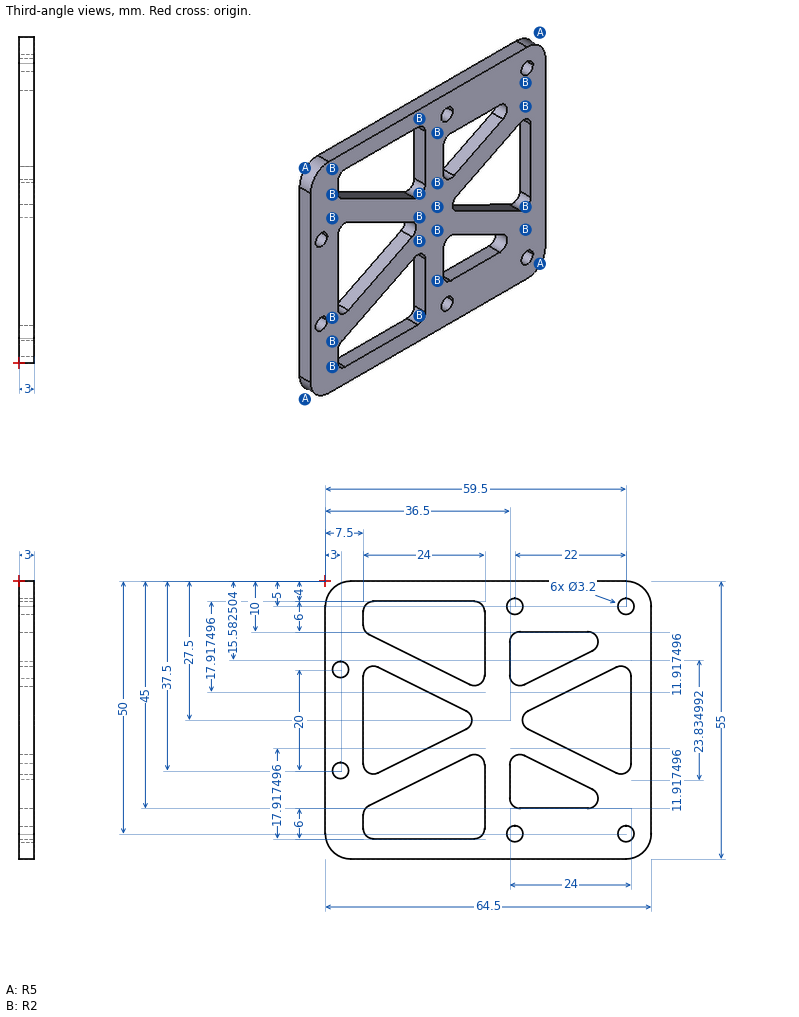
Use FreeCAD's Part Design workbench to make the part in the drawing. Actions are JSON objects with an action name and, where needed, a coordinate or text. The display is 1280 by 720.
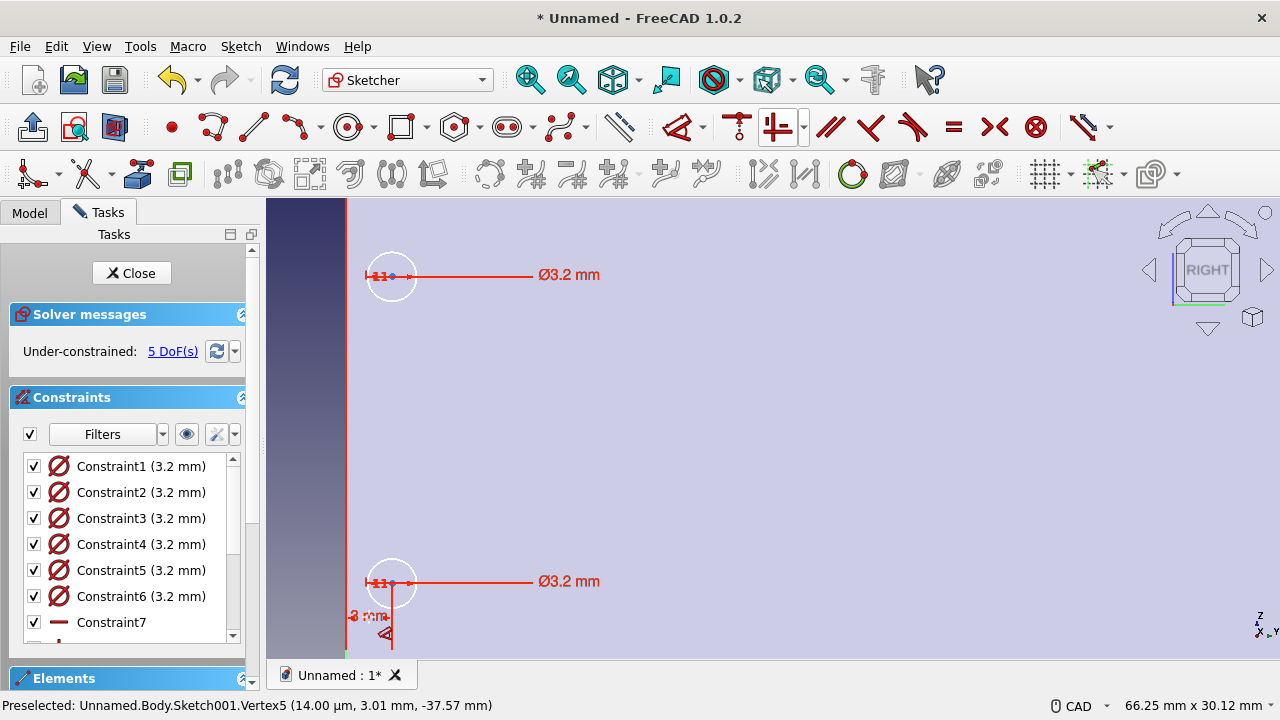
{"action": "scroll", "coordinate": [641, 443], "scroll_direction": "down", "scroll_amount": 5}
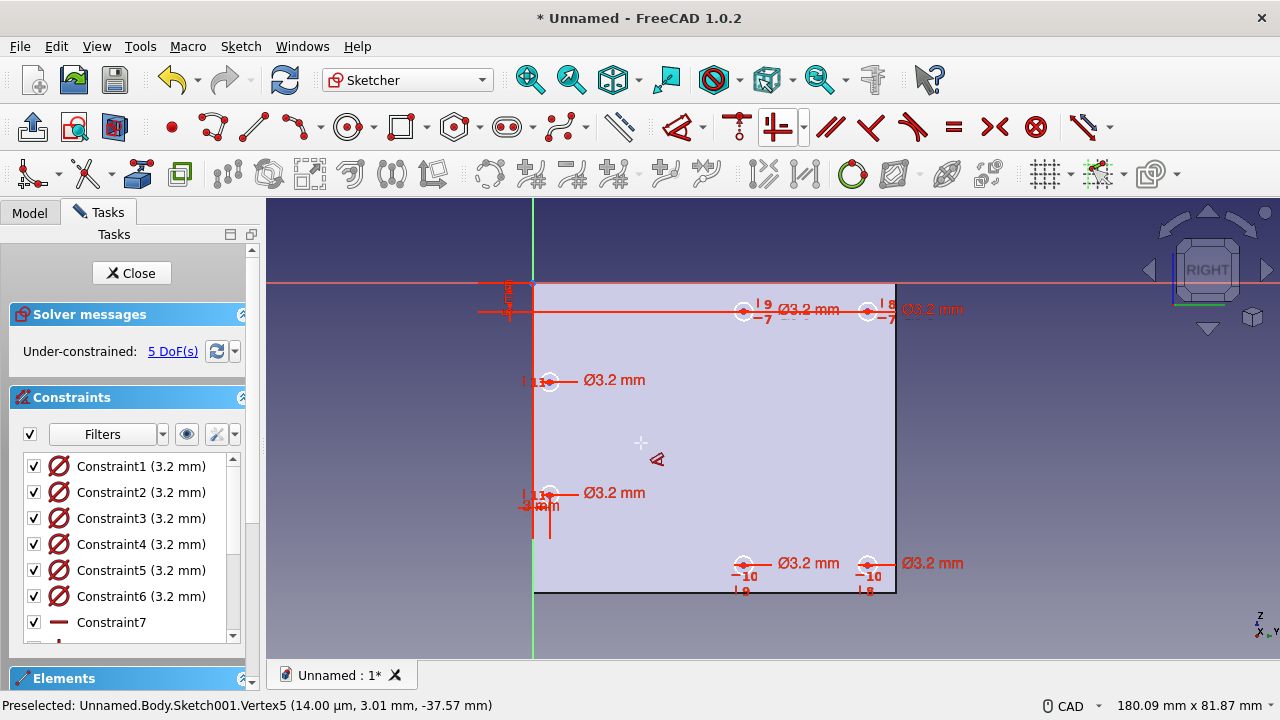
{"action": "left_click", "coordinate": [868, 565]}
{"action": "left_click", "coordinate": [499, 424]}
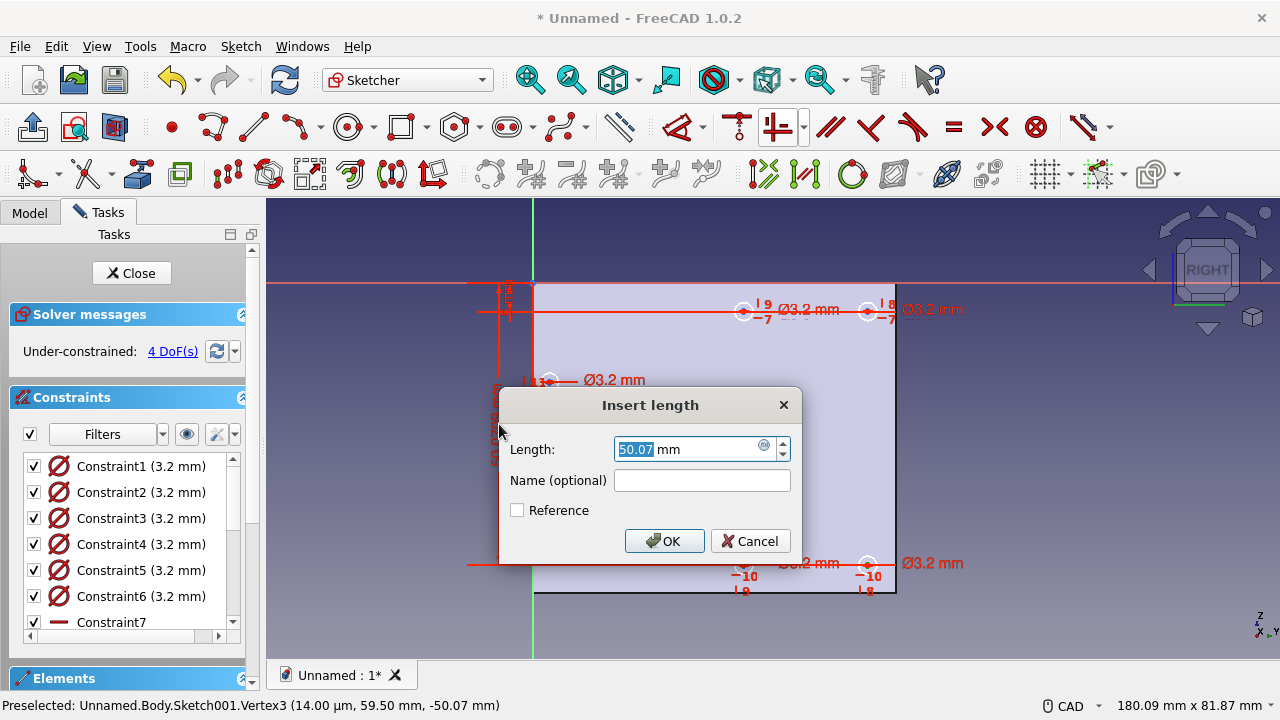
{"action": "type", "text": "50"}
{"action": "key", "text": "Return"}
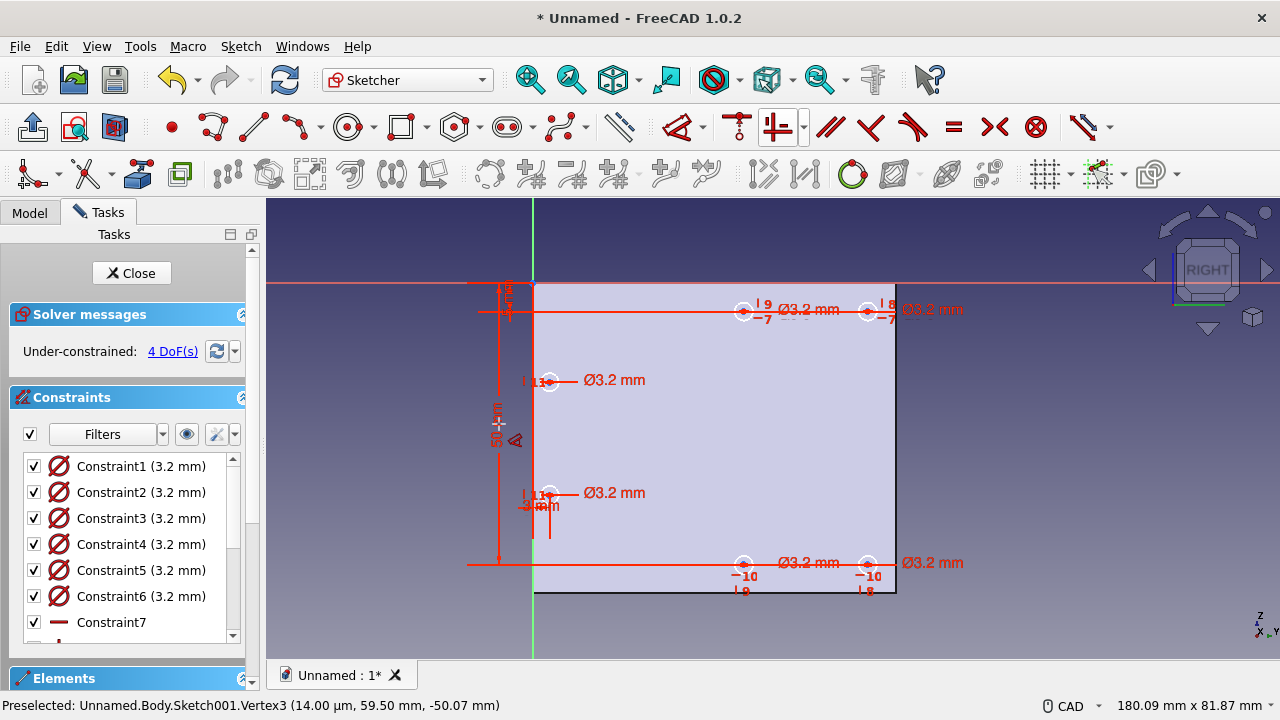
{"action": "left_click", "coordinate": [868, 312]}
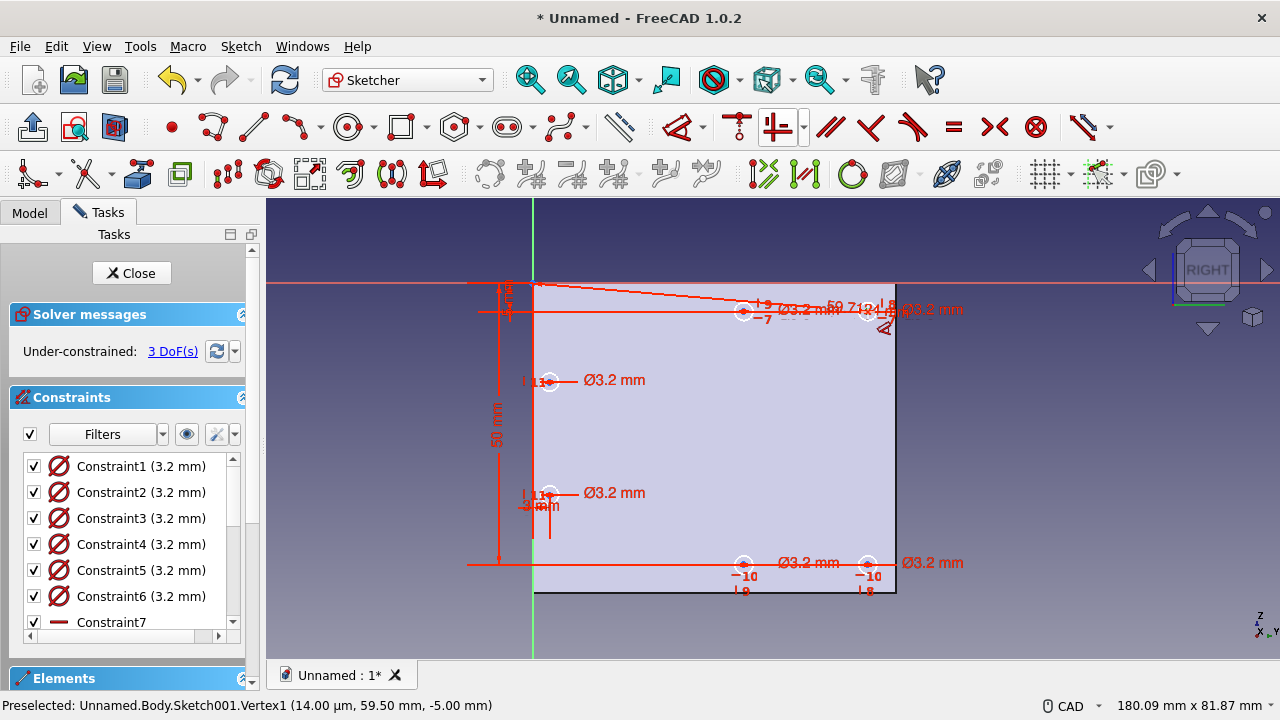
{"action": "left_click", "coordinate": [744, 312]}
{"action": "left_click", "coordinate": [806, 346]}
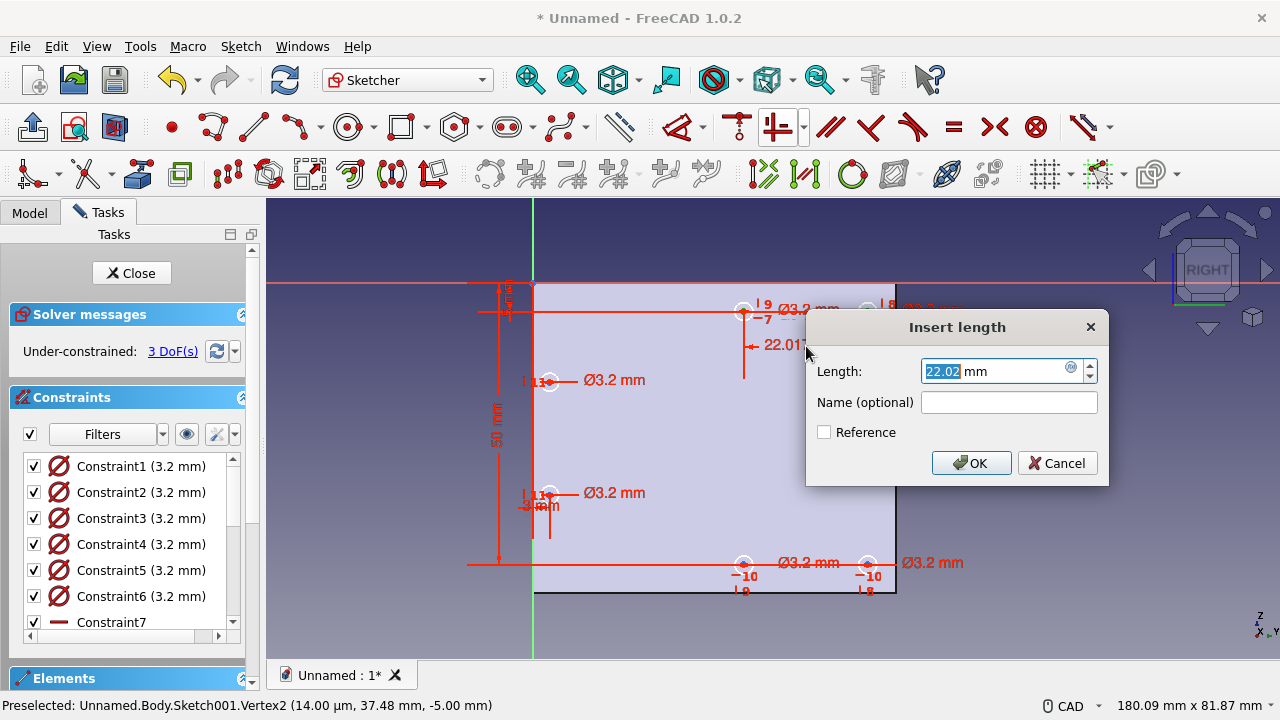
{"action": "type", "text": "22"}
{"action": "key", "text": "Return"}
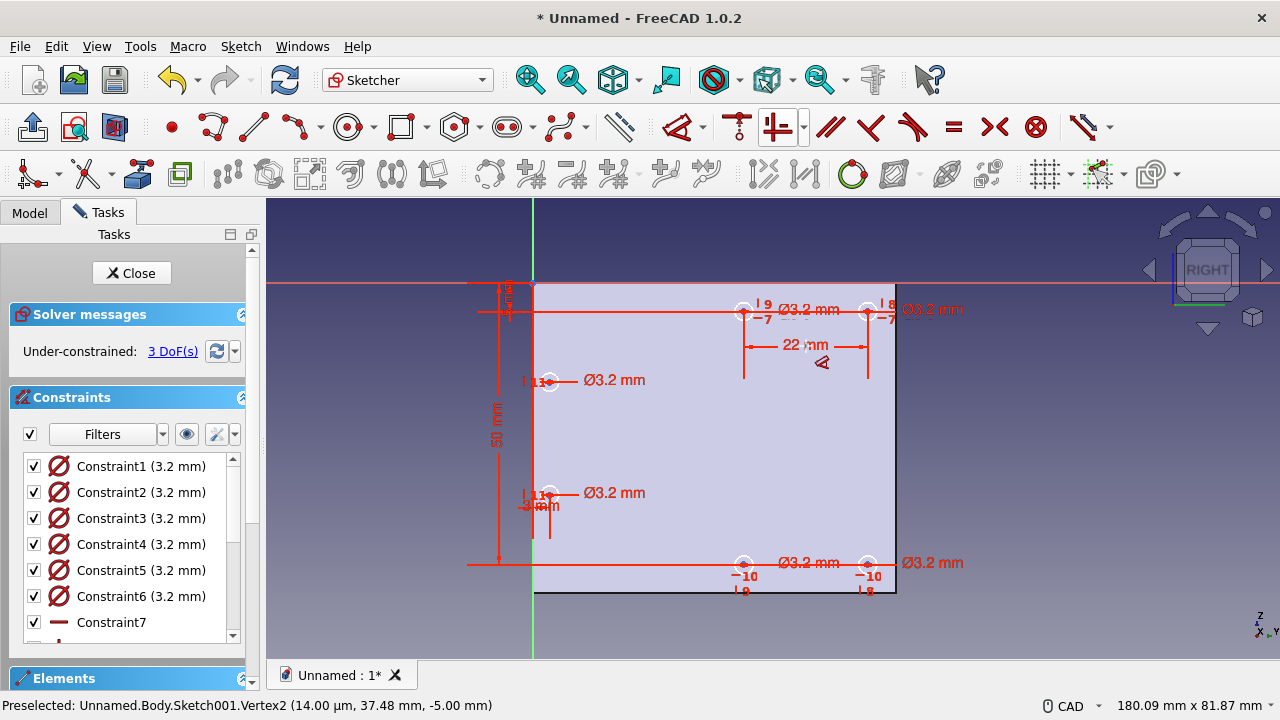
{"action": "left_click", "coordinate": [550, 495]}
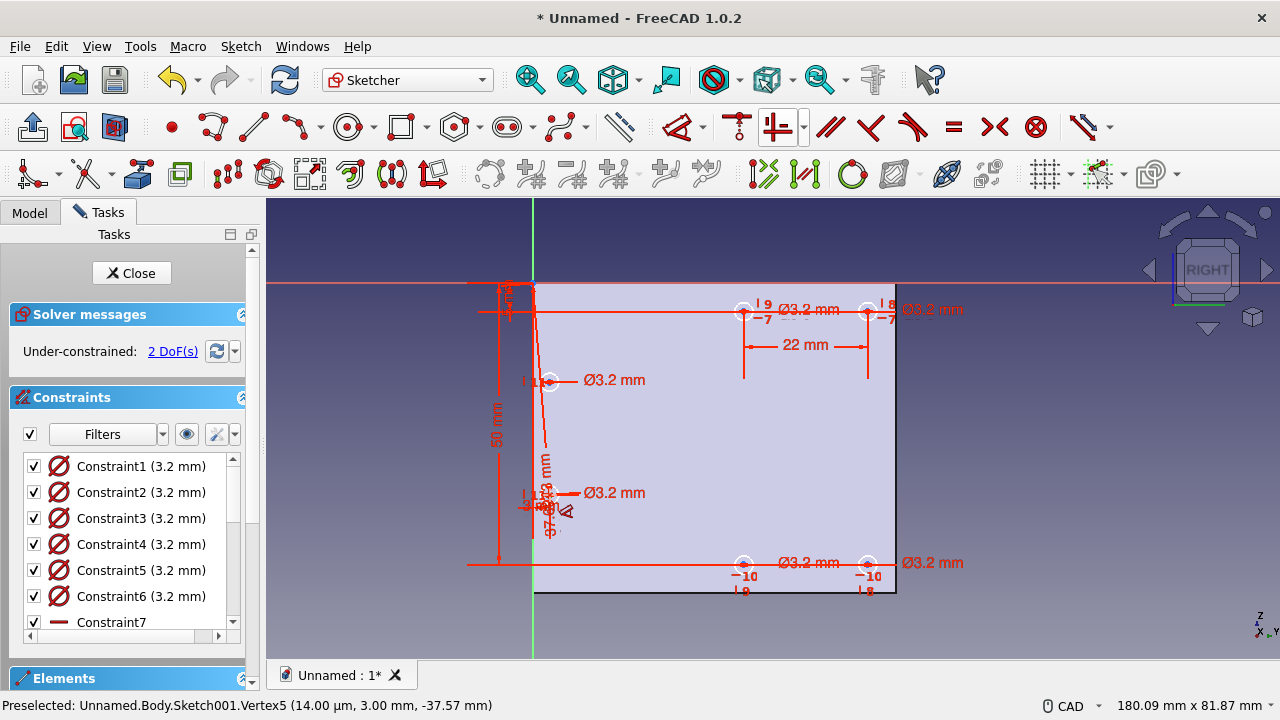
{"action": "left_click", "coordinate": [550, 382]}
{"action": "left_click", "coordinate": [516, 465]}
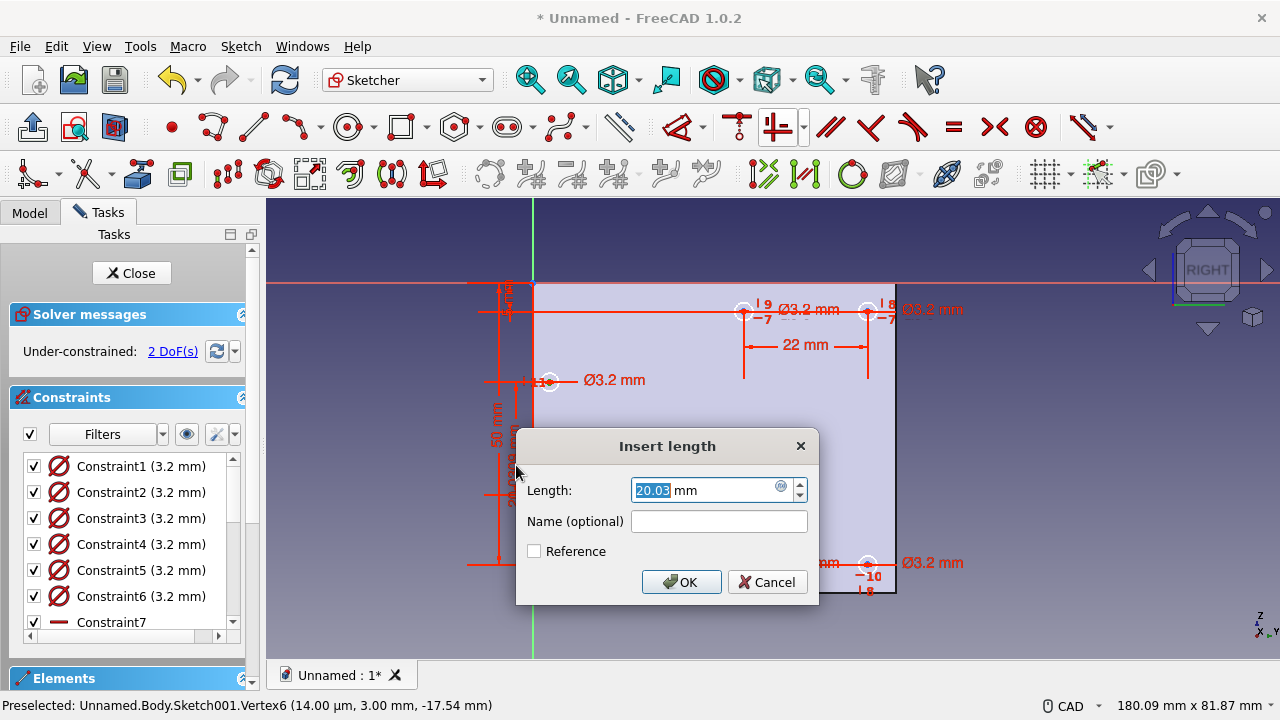
{"action": "type", "text": "20"}
{"action": "key", "text": "Return"}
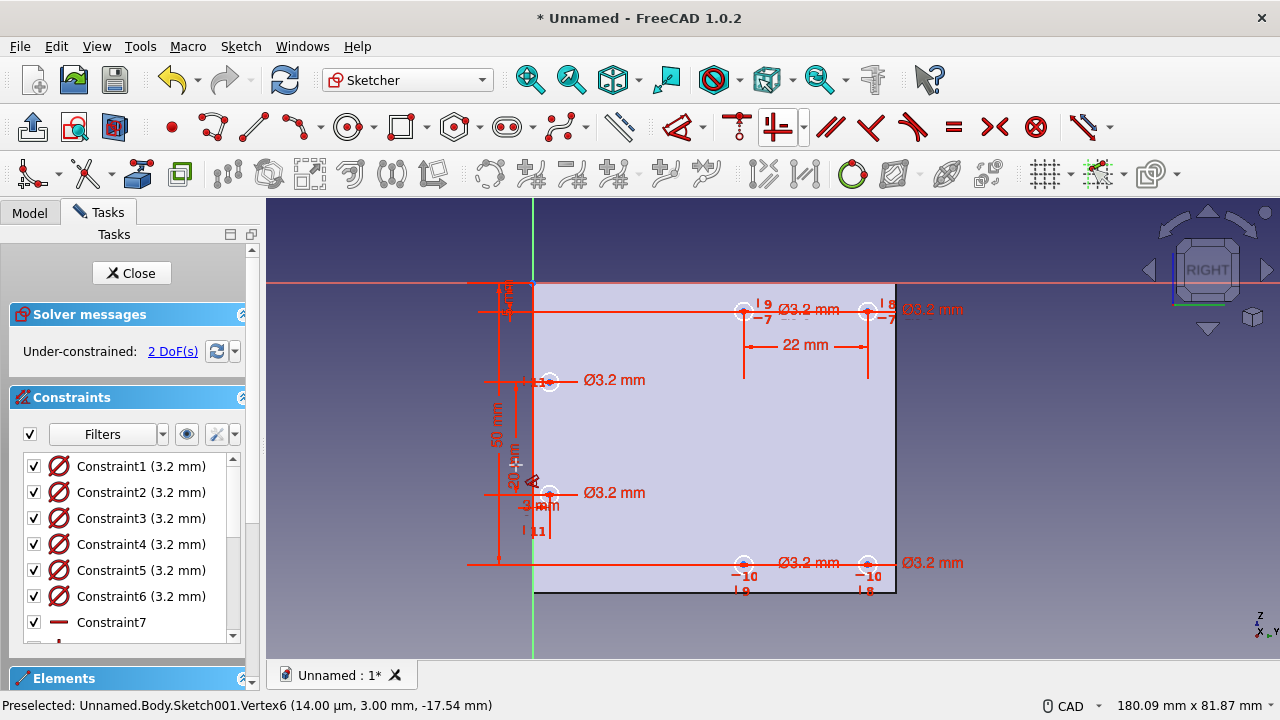
{"action": "left_click", "coordinate": [868, 312]}
{"action": "left_click", "coordinate": [700, 249]}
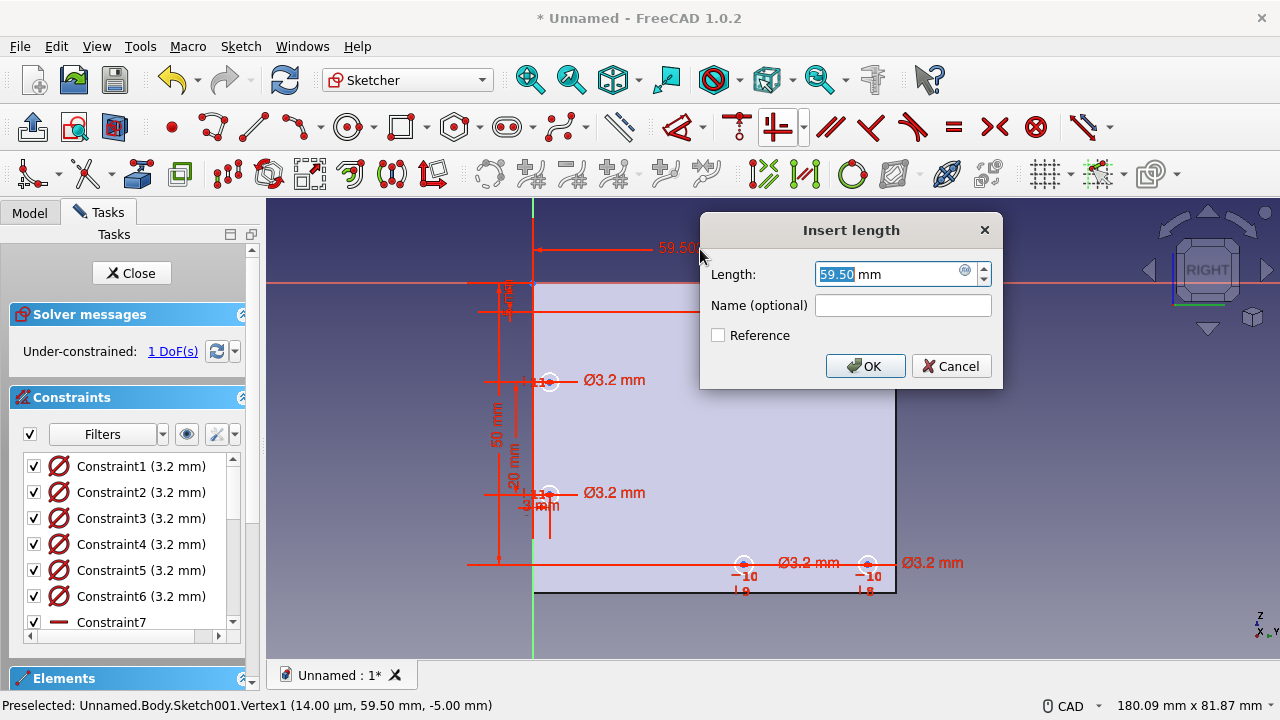
{"action": "type", "text": "59.5"}
{"action": "key", "text": "Return"}